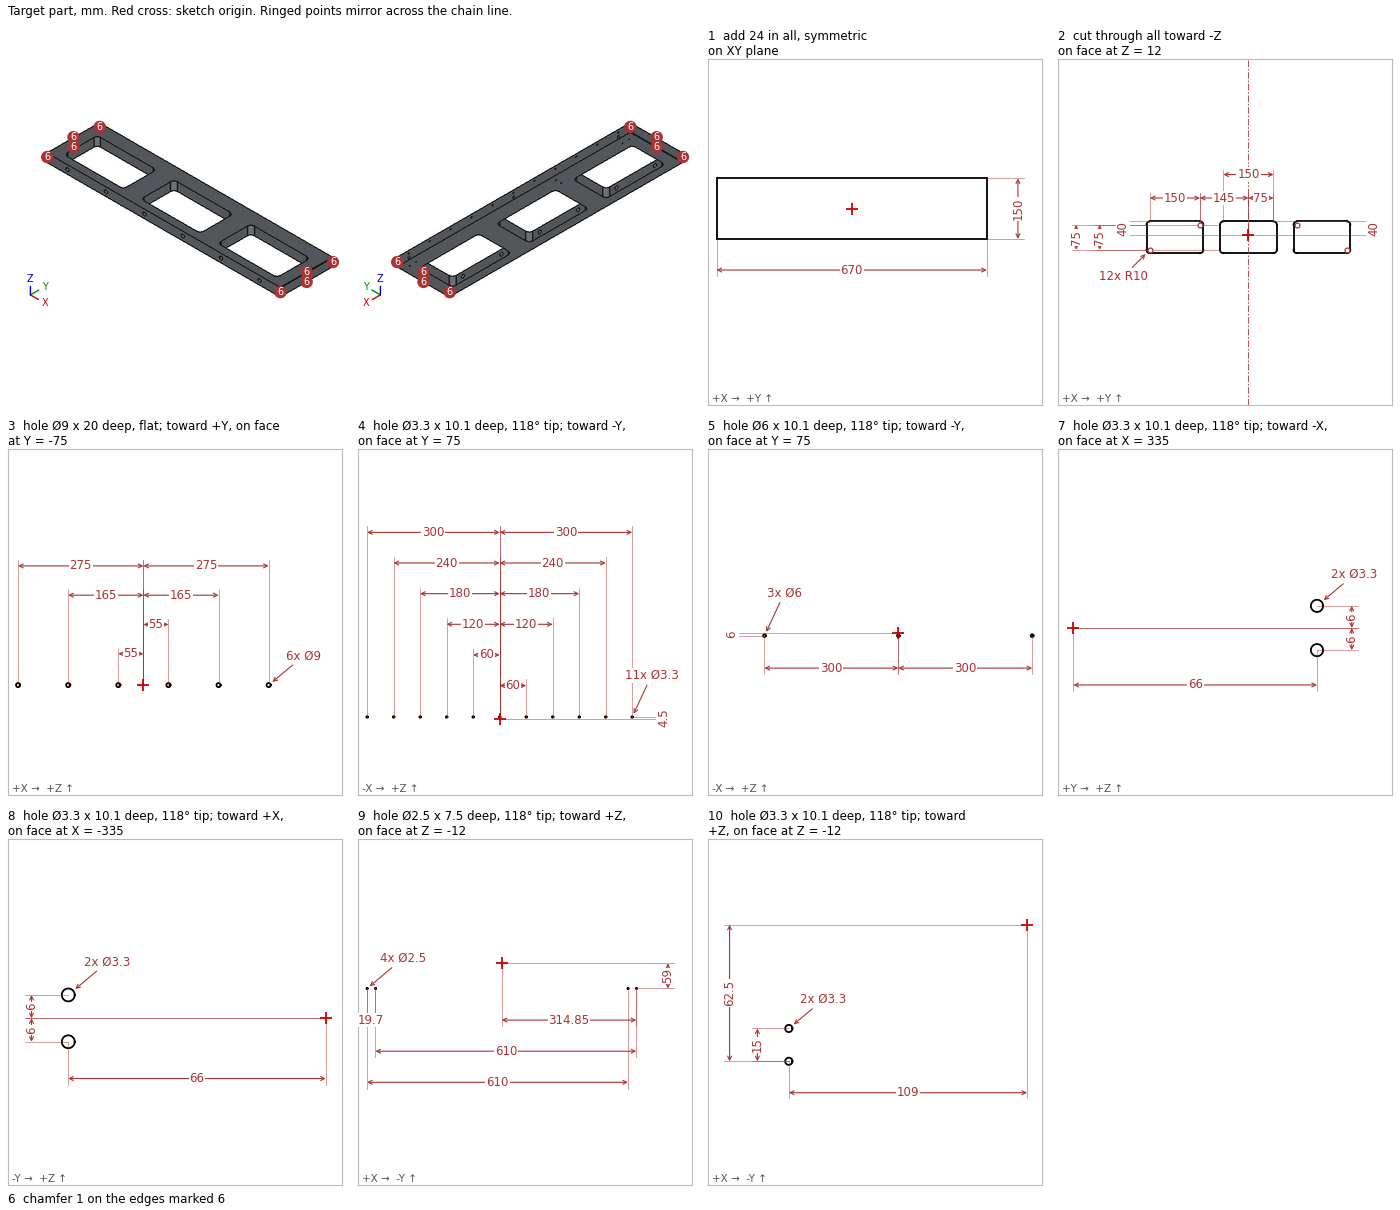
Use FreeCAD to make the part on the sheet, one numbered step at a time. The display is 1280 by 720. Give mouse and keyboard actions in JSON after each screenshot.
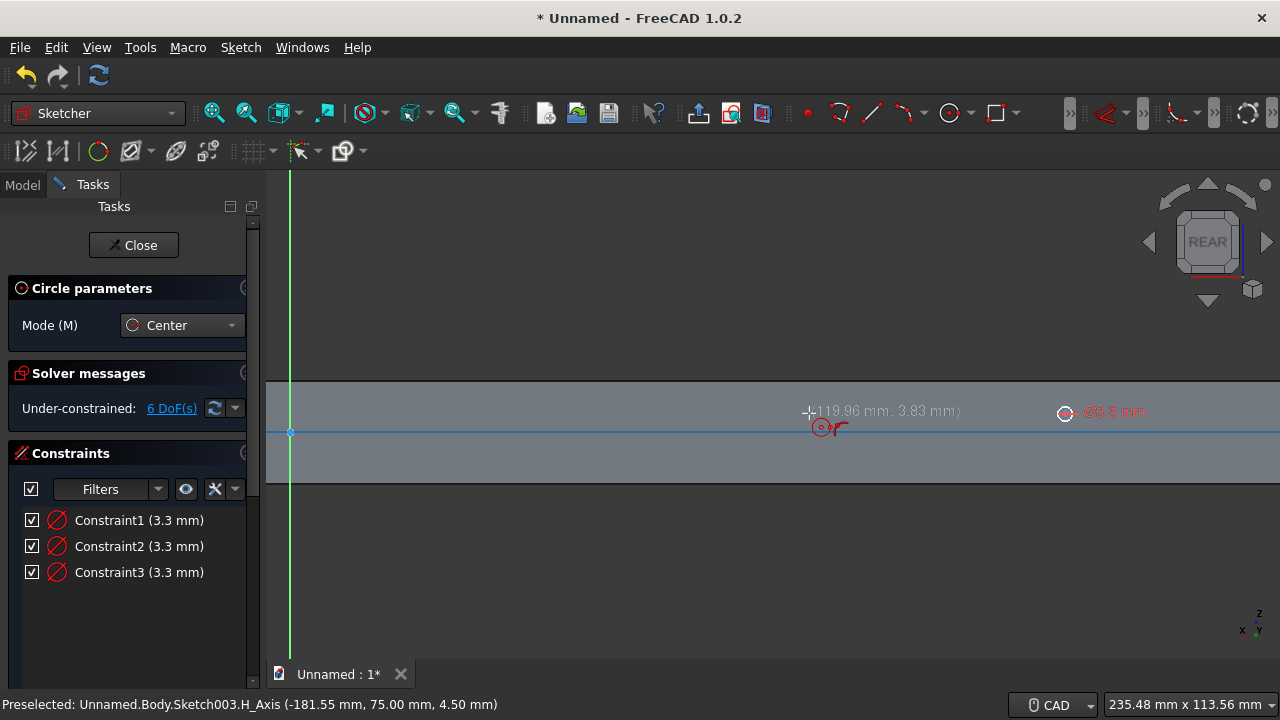
{"action": "left_click", "coordinate": [807, 413]}
{"action": "mouse_move", "coordinate": [812, 408]}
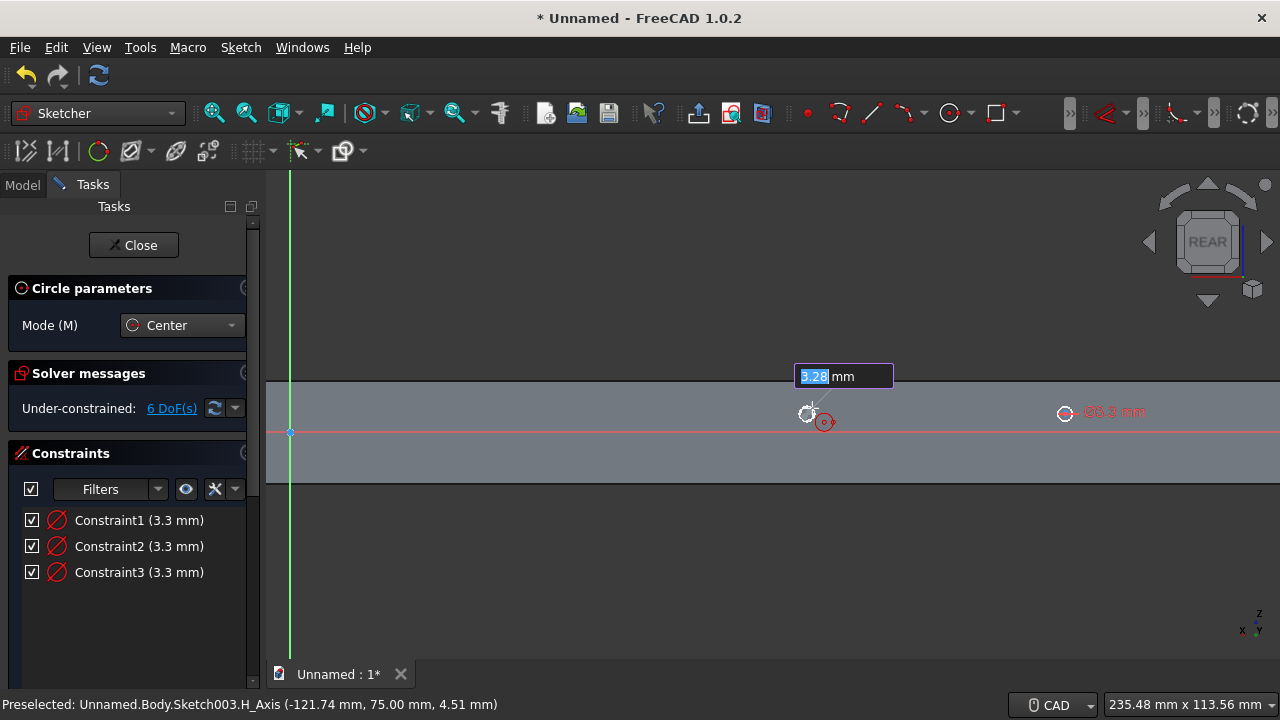
{"action": "type", "text": "3.3"}
{"action": "key", "text": "Return"}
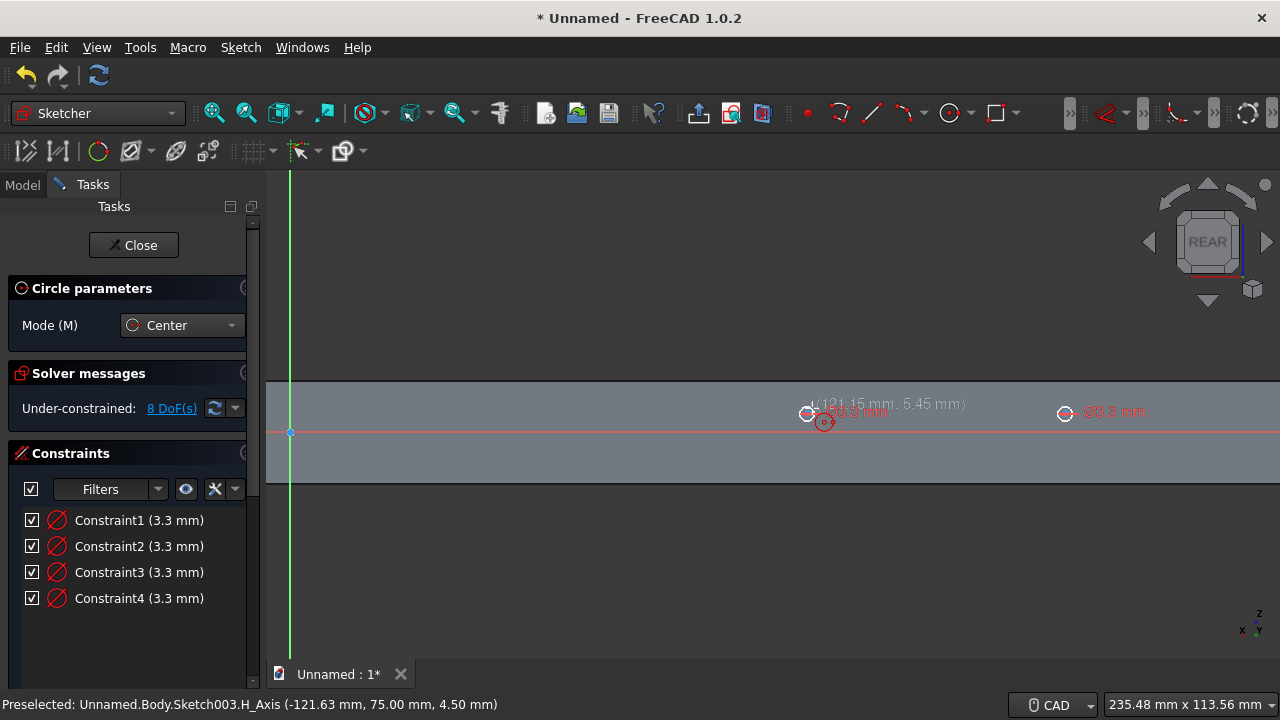
{"action": "scroll", "coordinate": [549, 413], "scroll_direction": "up", "scroll_amount": 6}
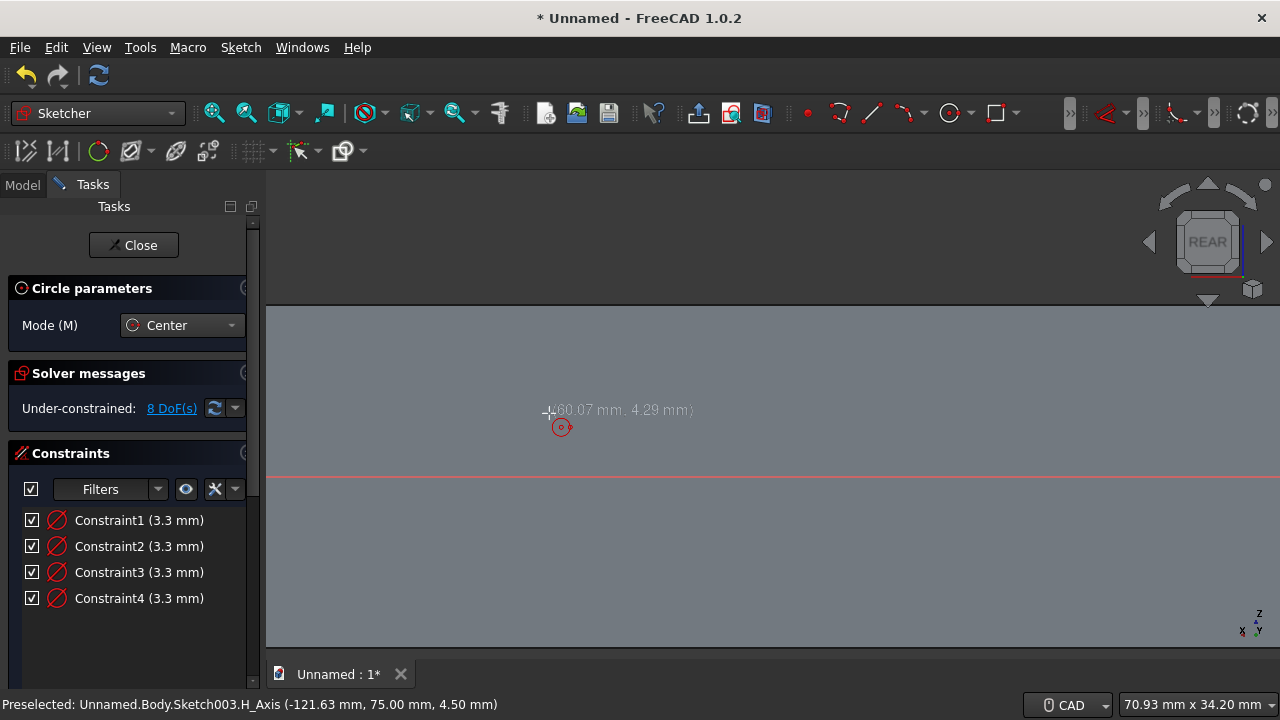
{"action": "scroll", "coordinate": [770, 413], "scroll_direction": "down", "scroll_amount": 14}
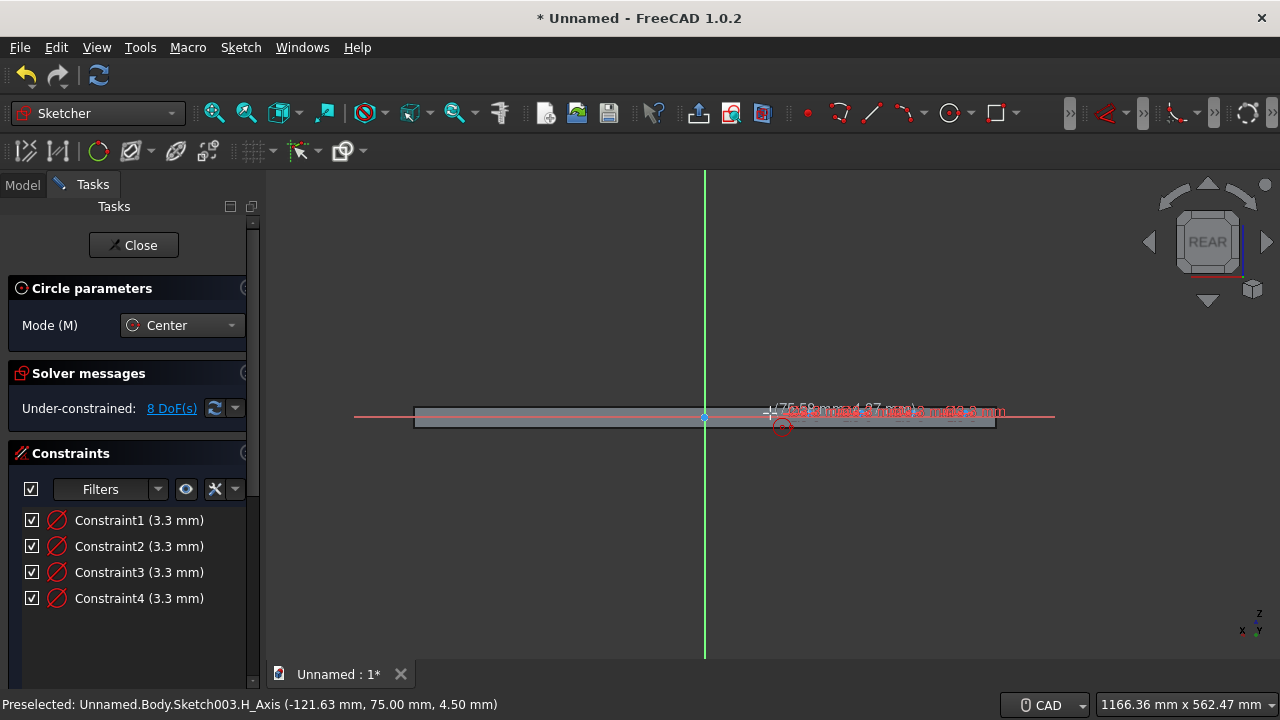
{"action": "scroll", "coordinate": [757, 413], "scroll_direction": "up", "scroll_amount": 8}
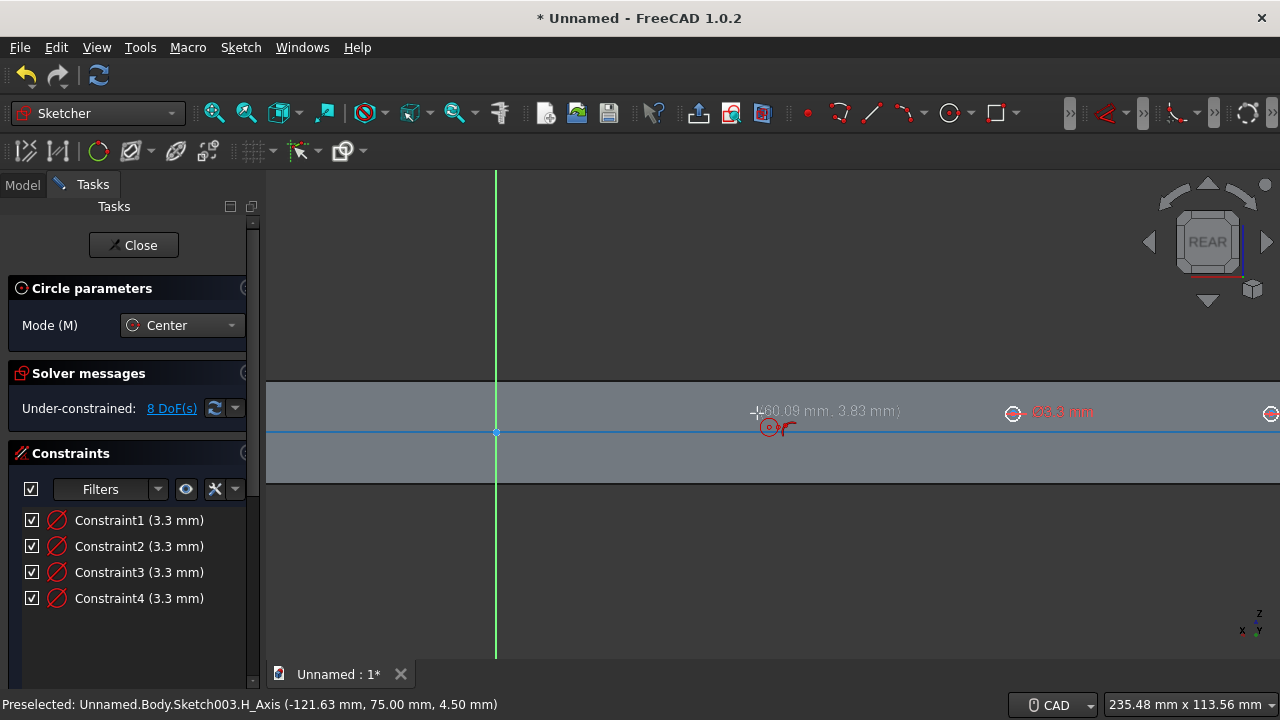
{"action": "left_click", "coordinate": [755, 413]}
{"action": "mouse_move", "coordinate": [760, 408]}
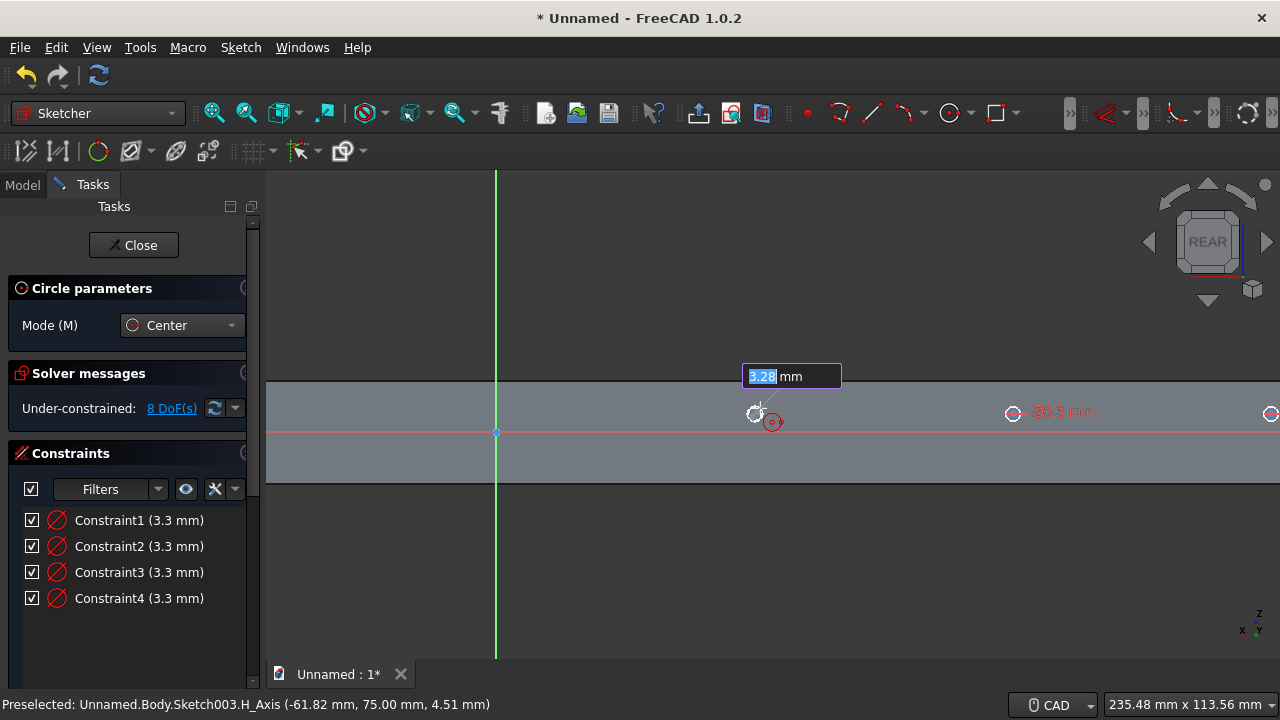
{"action": "type", "text": "3.3"}
{"action": "key", "text": "Return"}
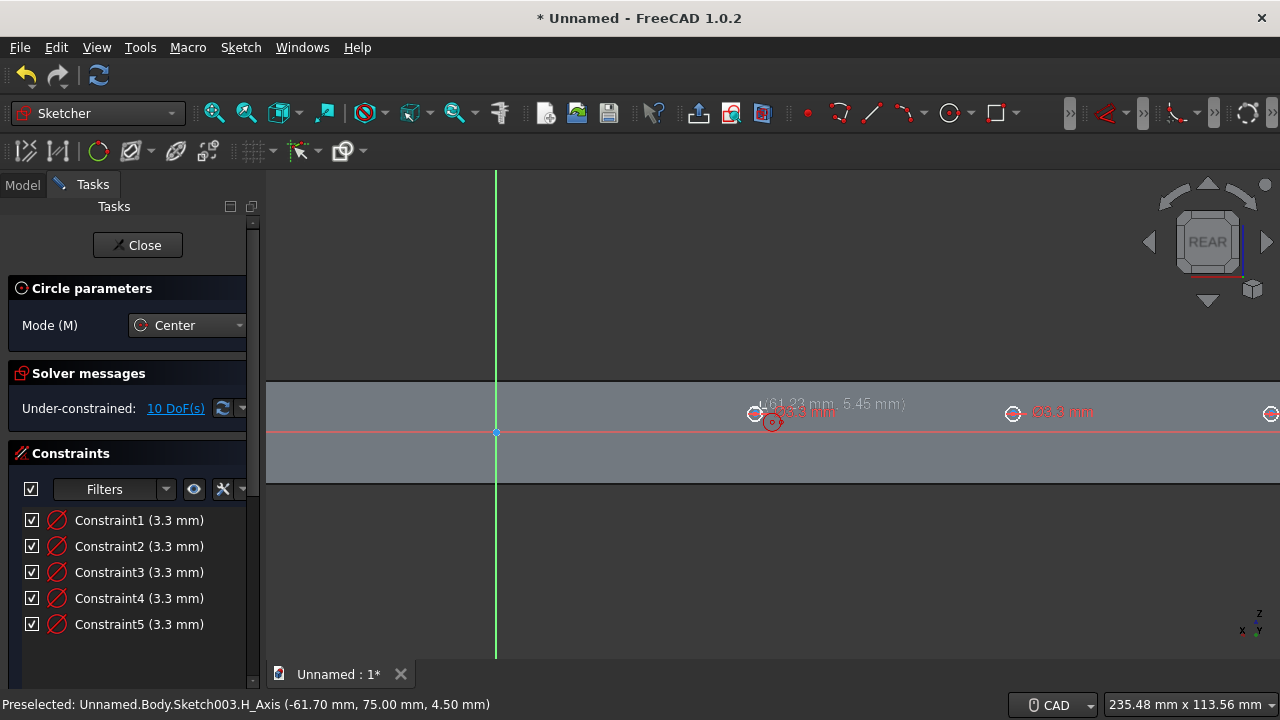
{"action": "scroll", "coordinate": [496, 413], "scroll_direction": "up", "scroll_amount": 6}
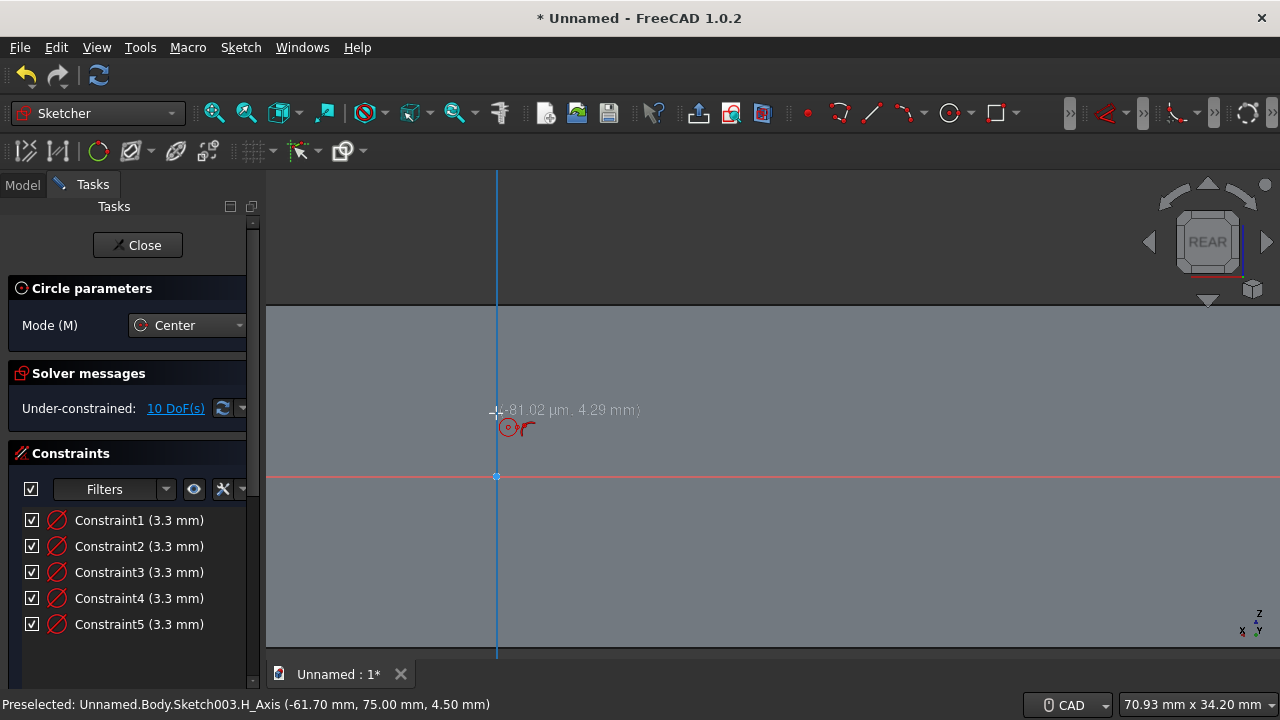
{"action": "scroll", "coordinate": [718, 413], "scroll_direction": "down", "scroll_amount": 14}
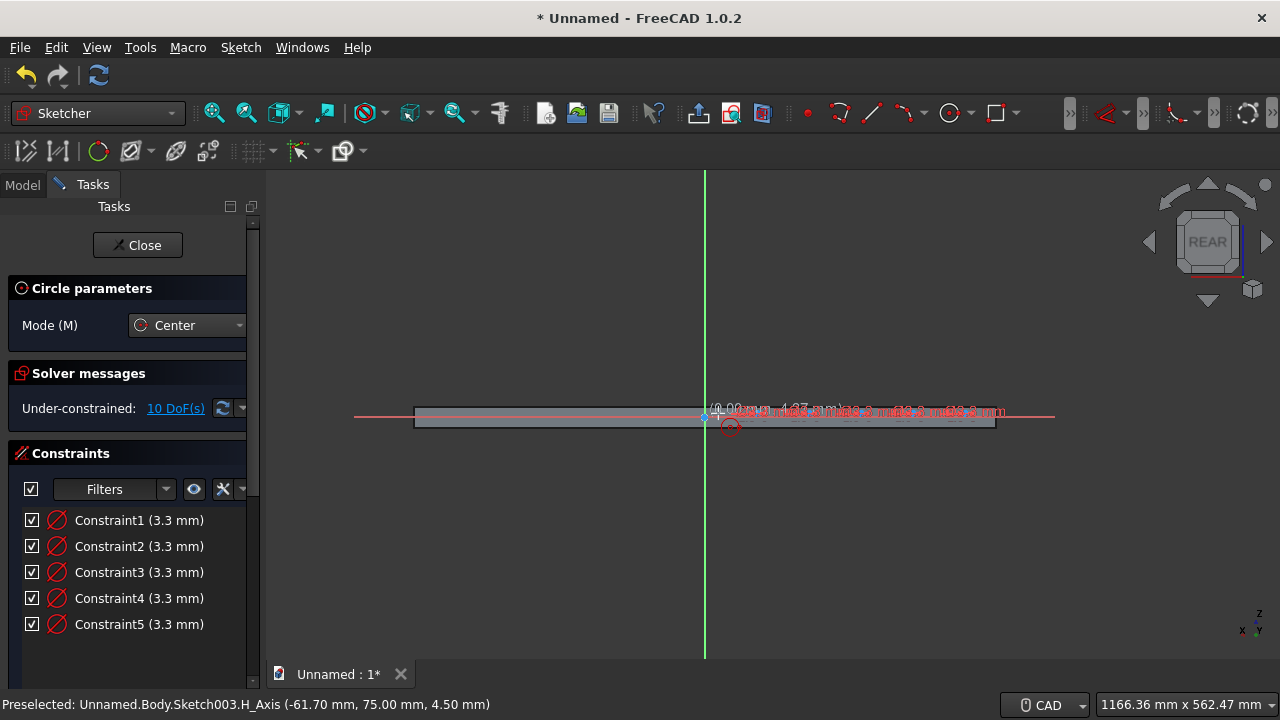
{"action": "scroll", "coordinate": [705, 413], "scroll_direction": "up", "scroll_amount": 8}